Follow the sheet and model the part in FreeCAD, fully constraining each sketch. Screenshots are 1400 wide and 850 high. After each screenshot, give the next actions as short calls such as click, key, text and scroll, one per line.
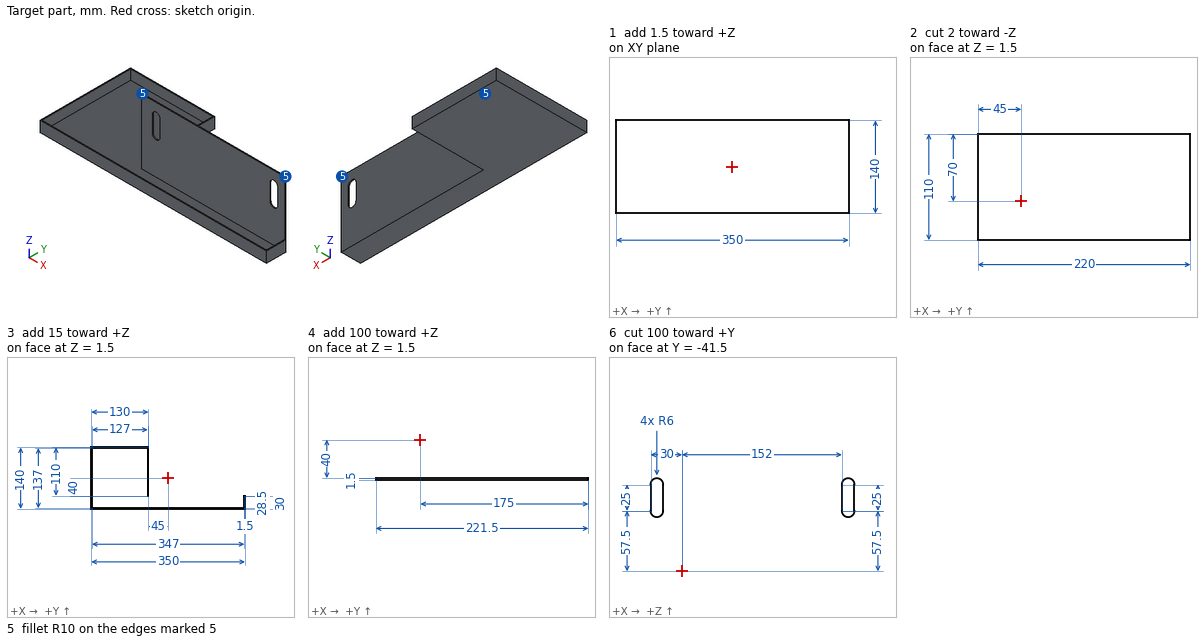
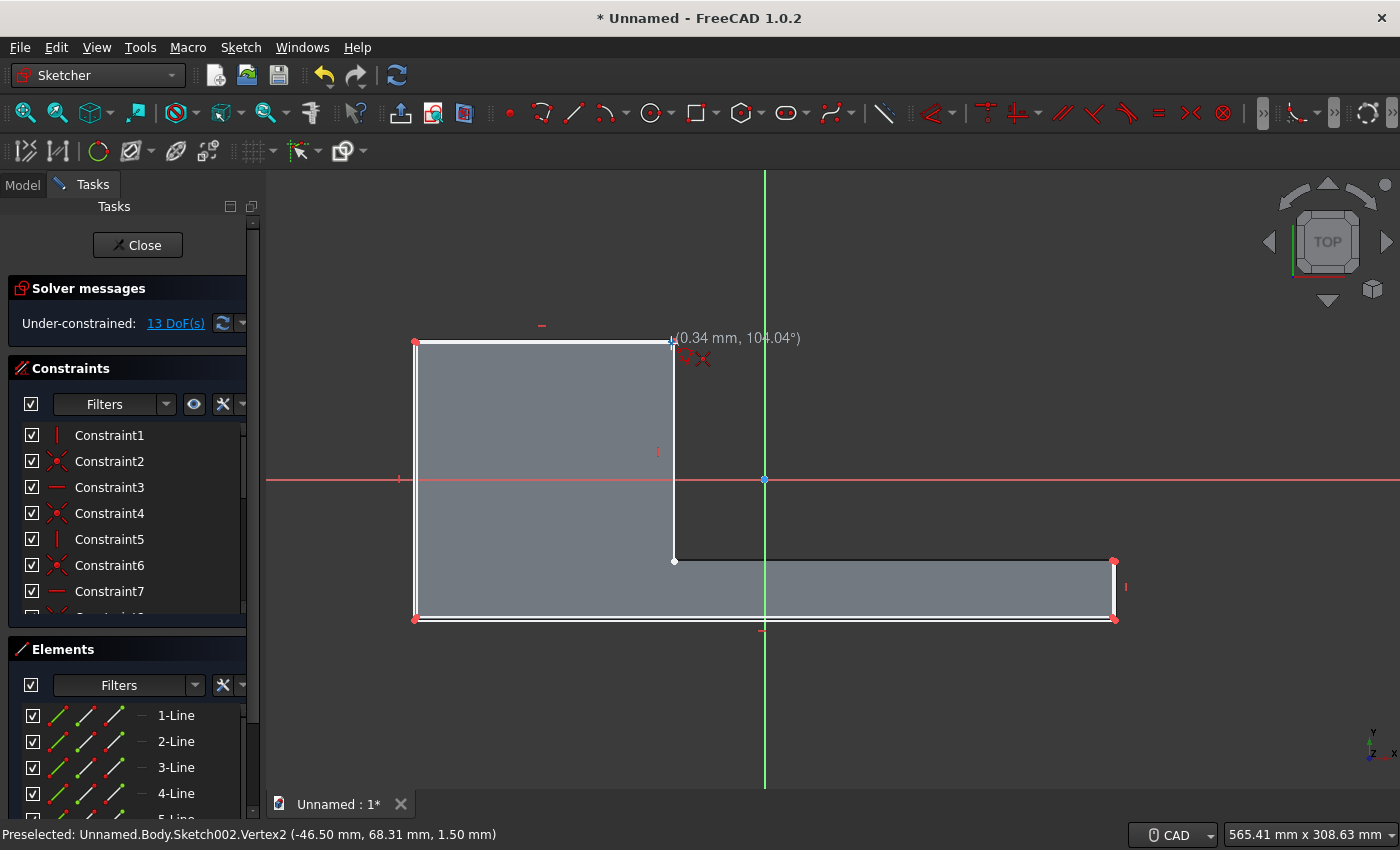
scroll(671, 560, up, 9)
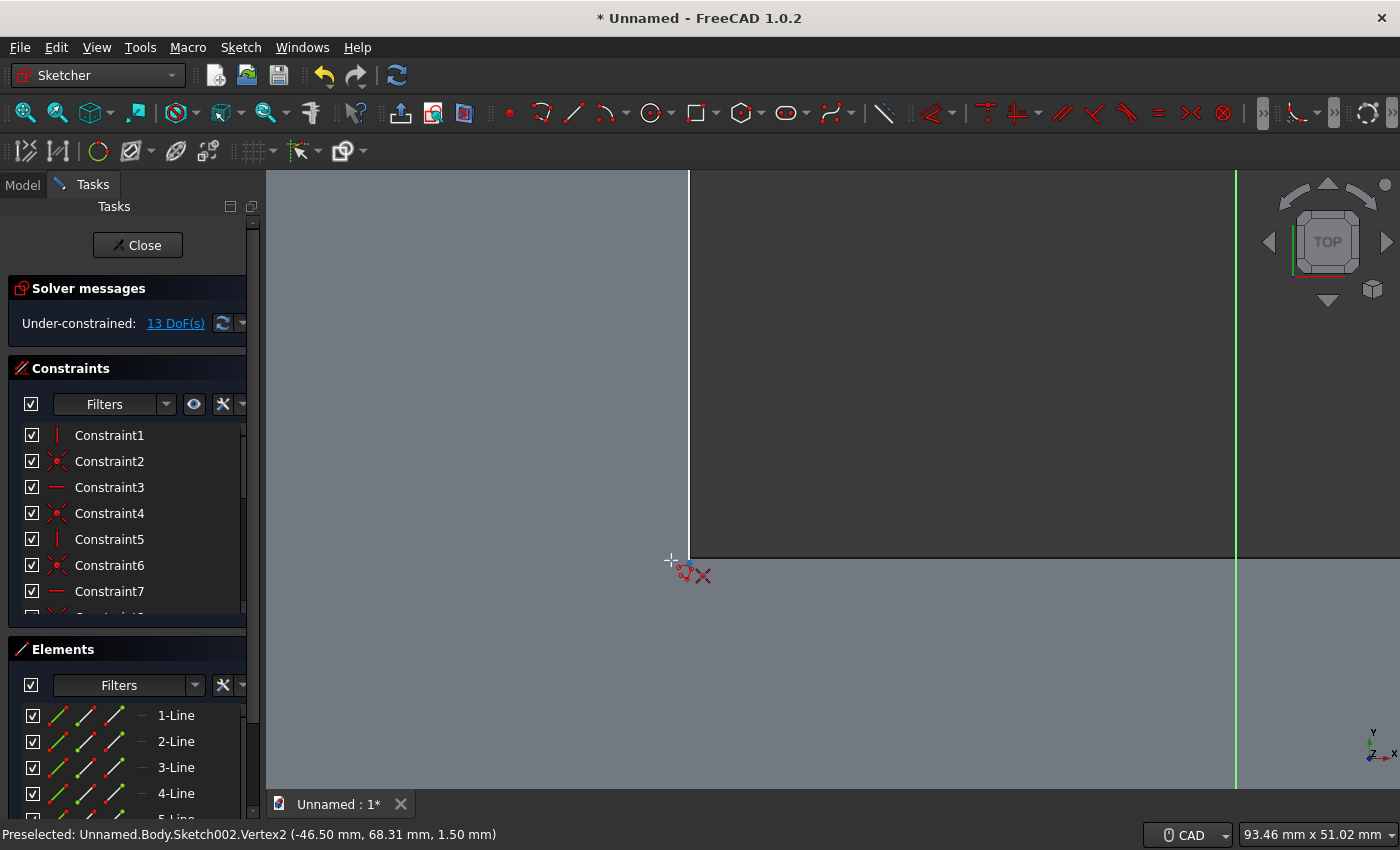
click(672, 558)
click(689, 564)
key(Escape)
key(Escape)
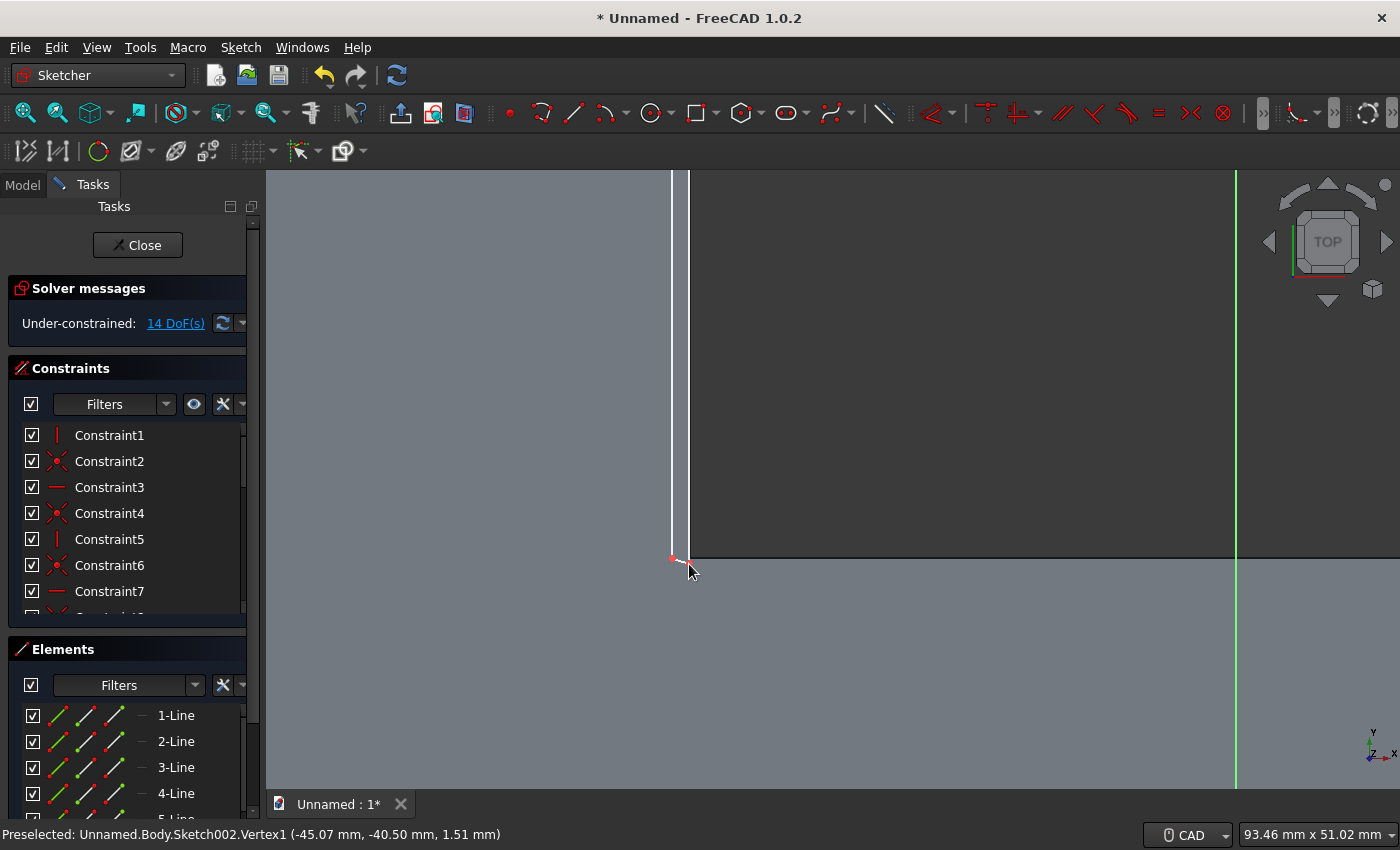
scroll(671, 560, down, 9)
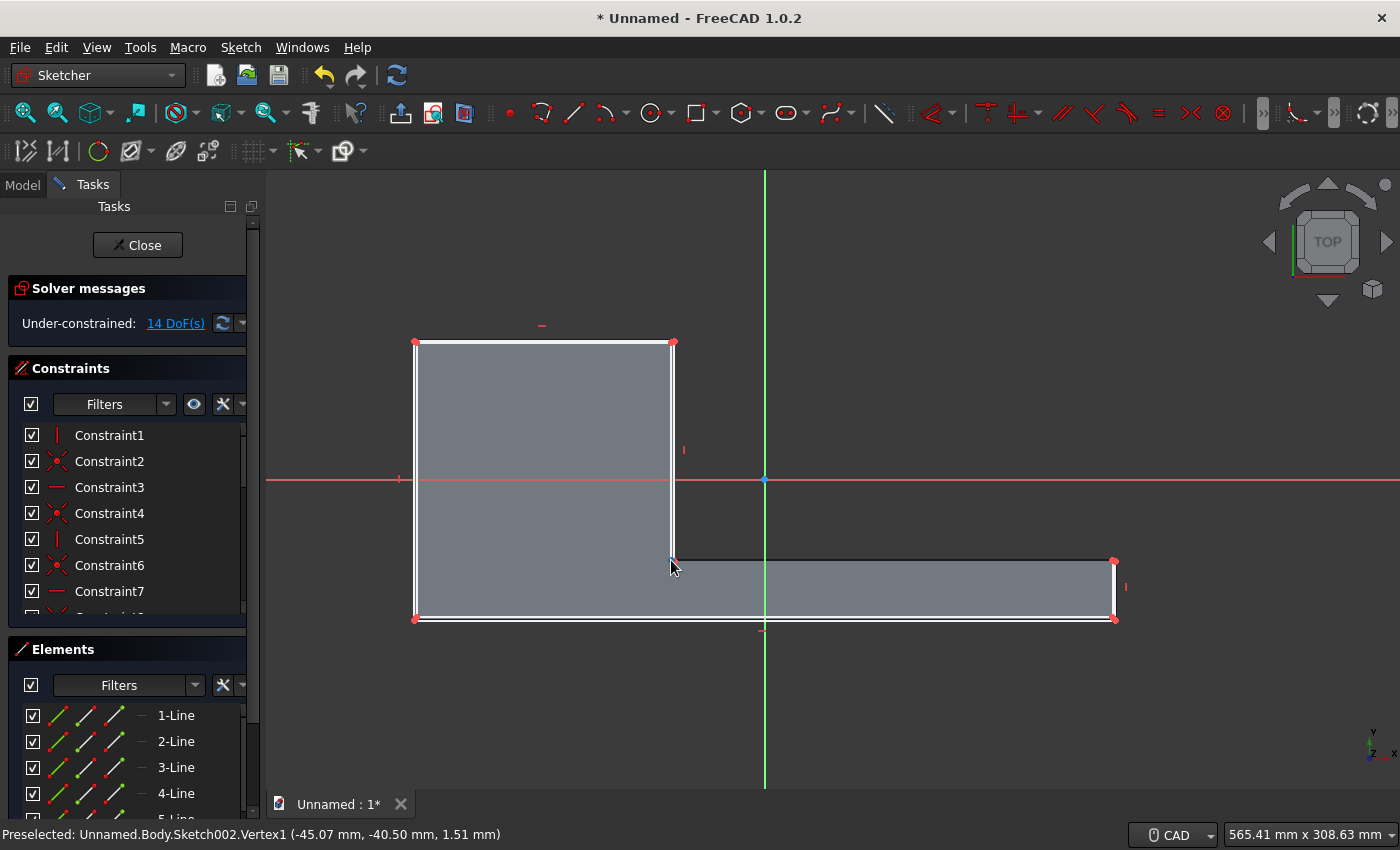
scroll(1114, 561, up, 12)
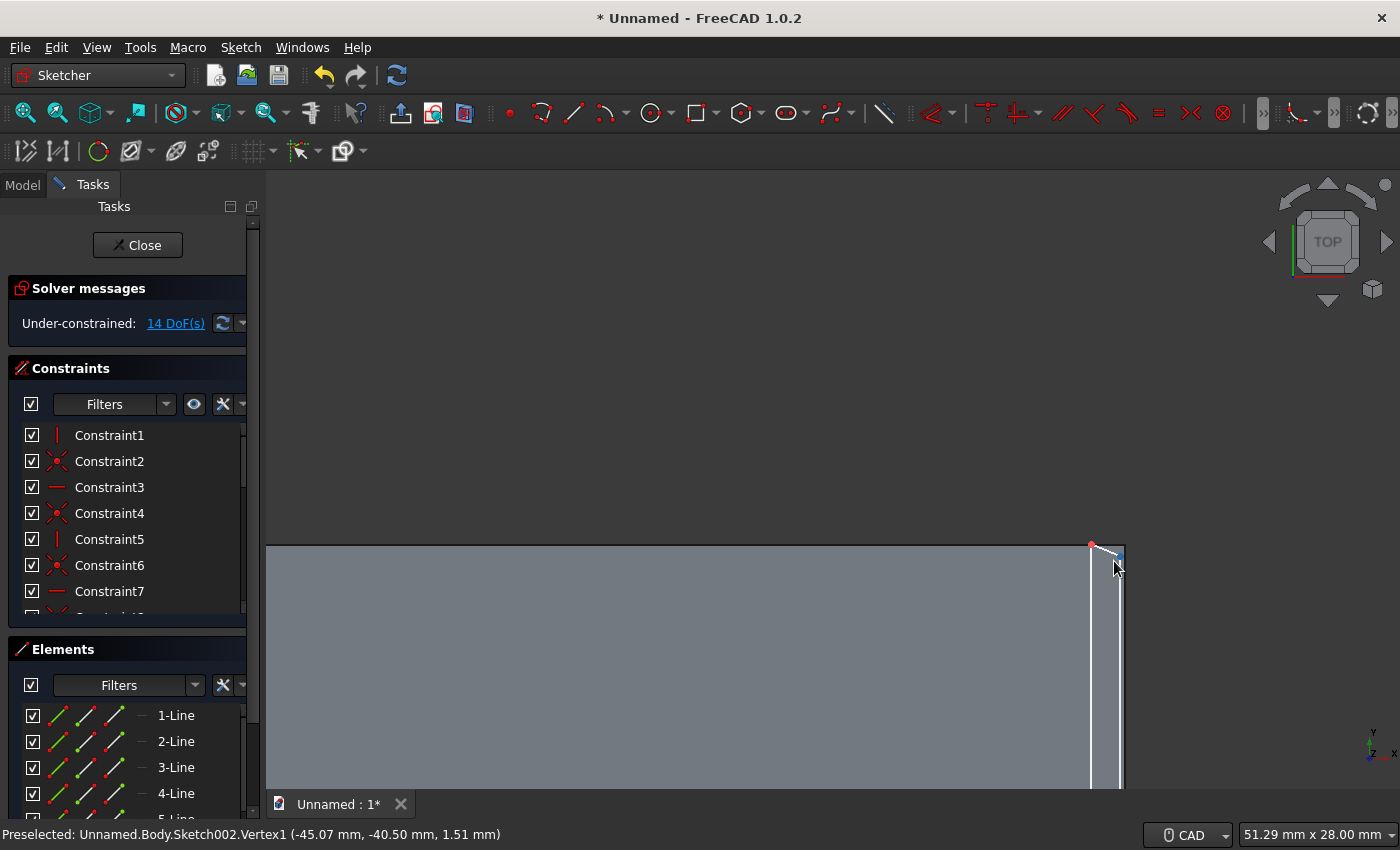
click(1106, 550)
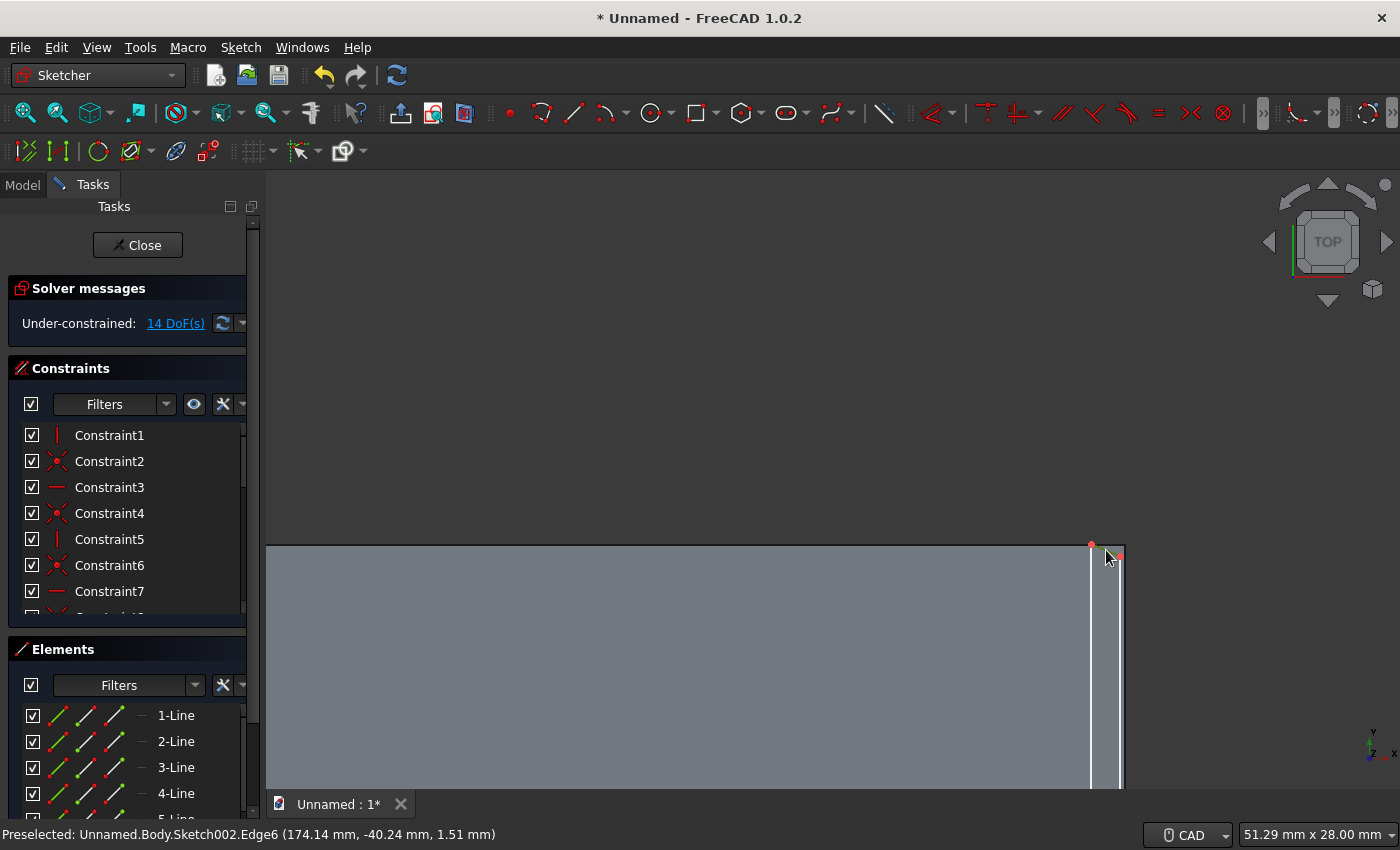
key(h)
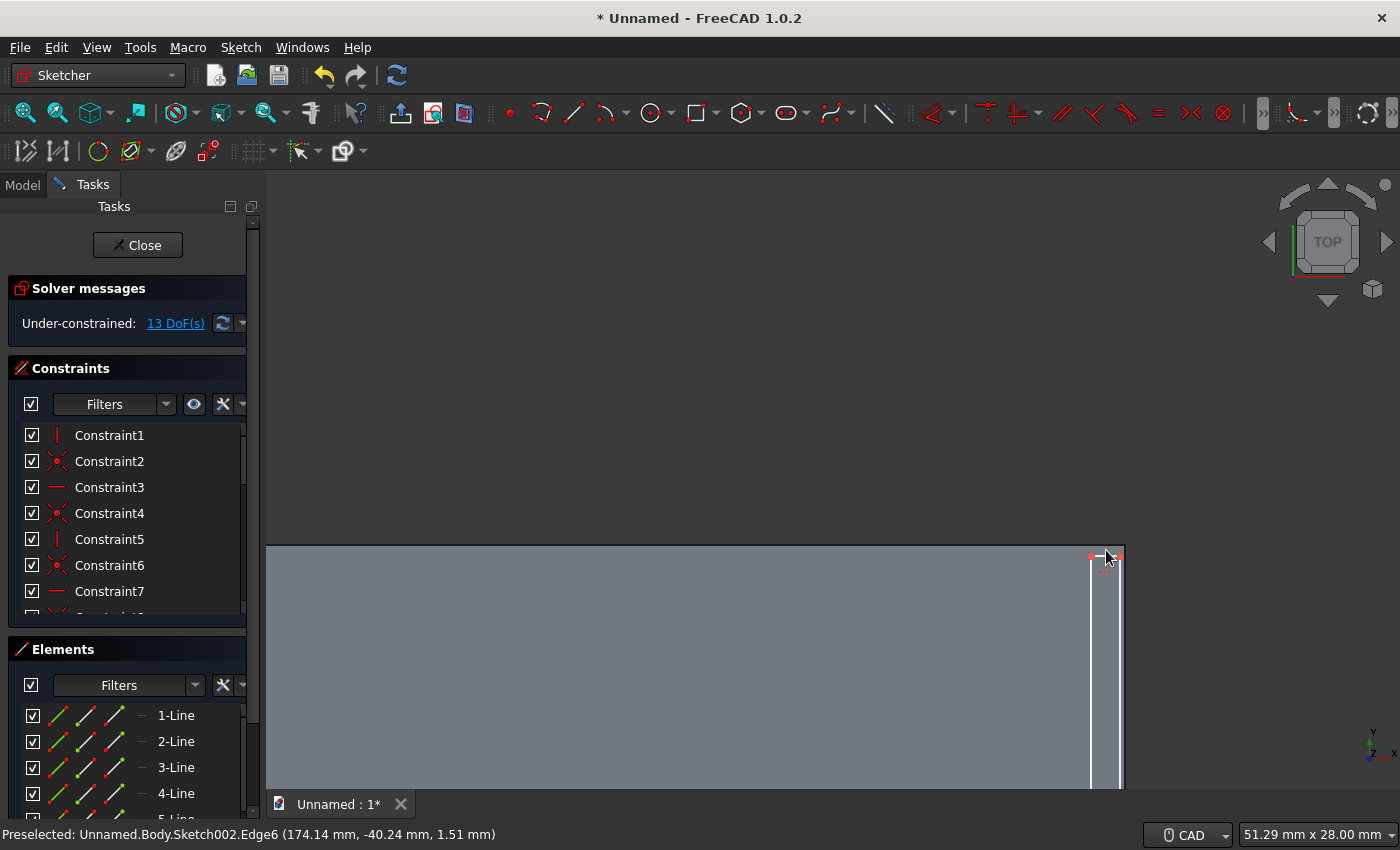
scroll(1115, 561, down, 12)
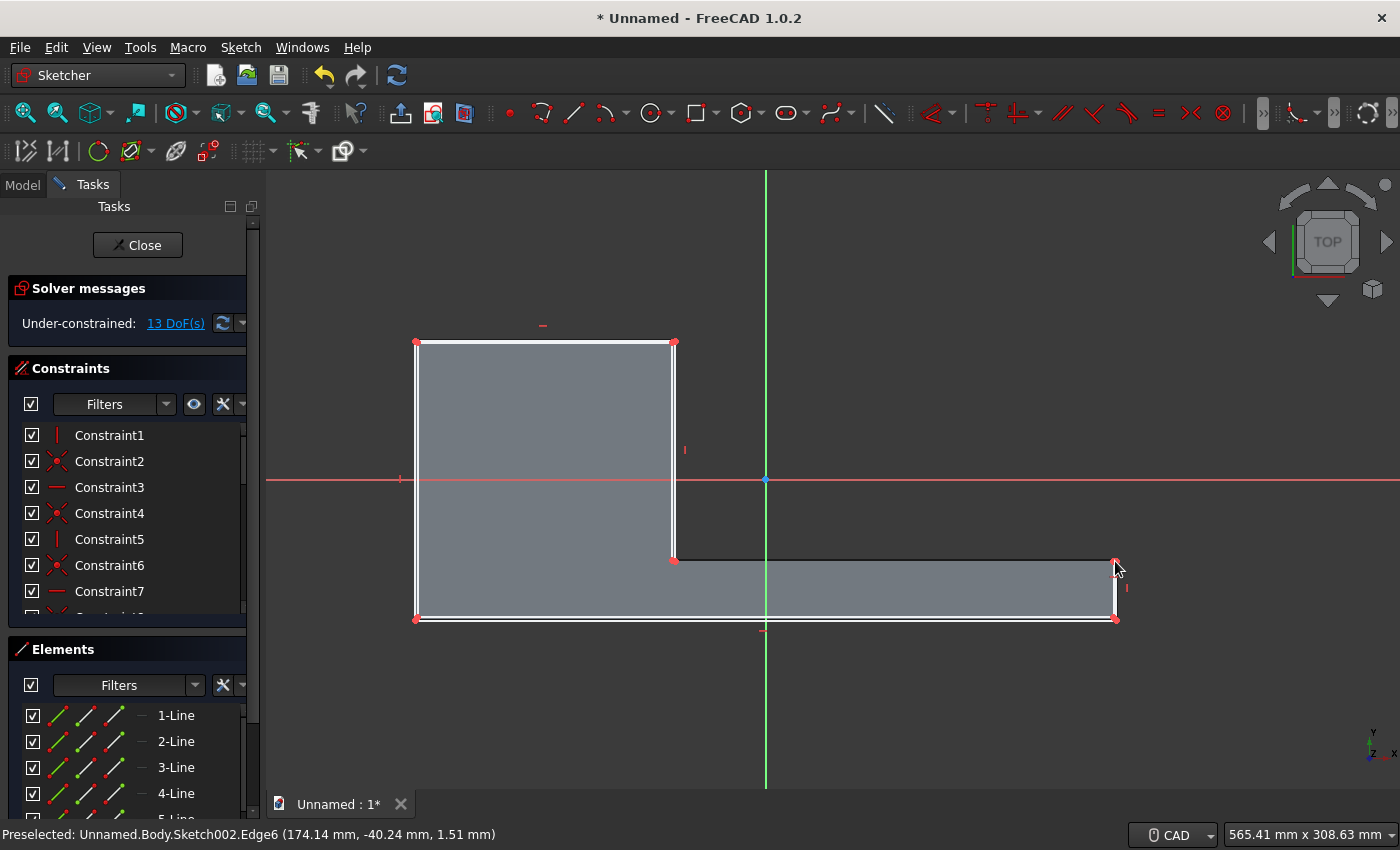
scroll(673, 561, up, 13)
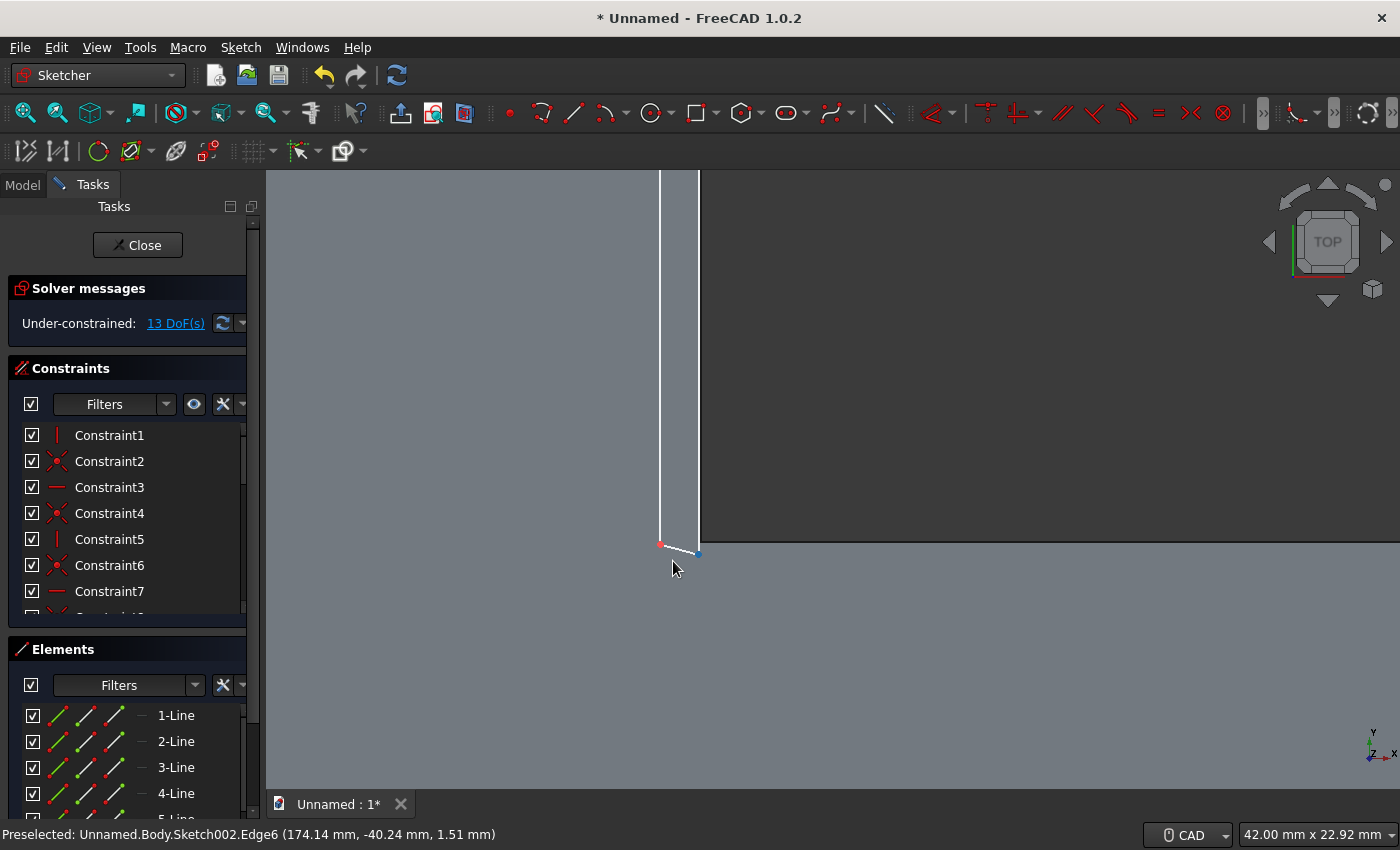
click(672, 548)